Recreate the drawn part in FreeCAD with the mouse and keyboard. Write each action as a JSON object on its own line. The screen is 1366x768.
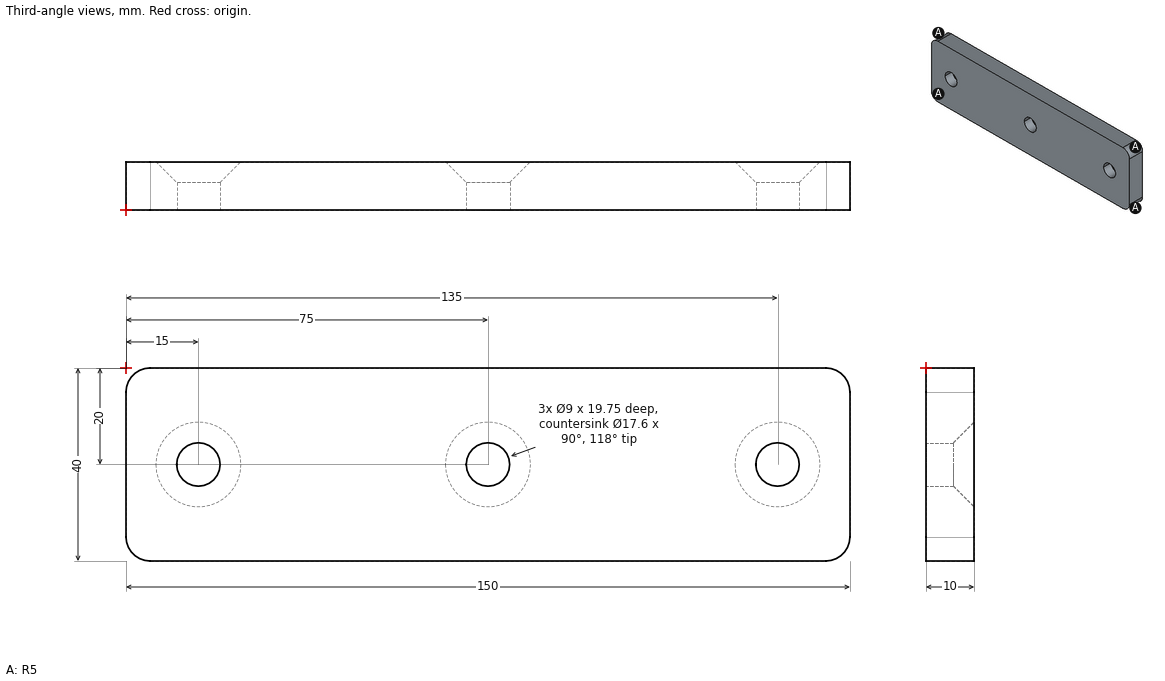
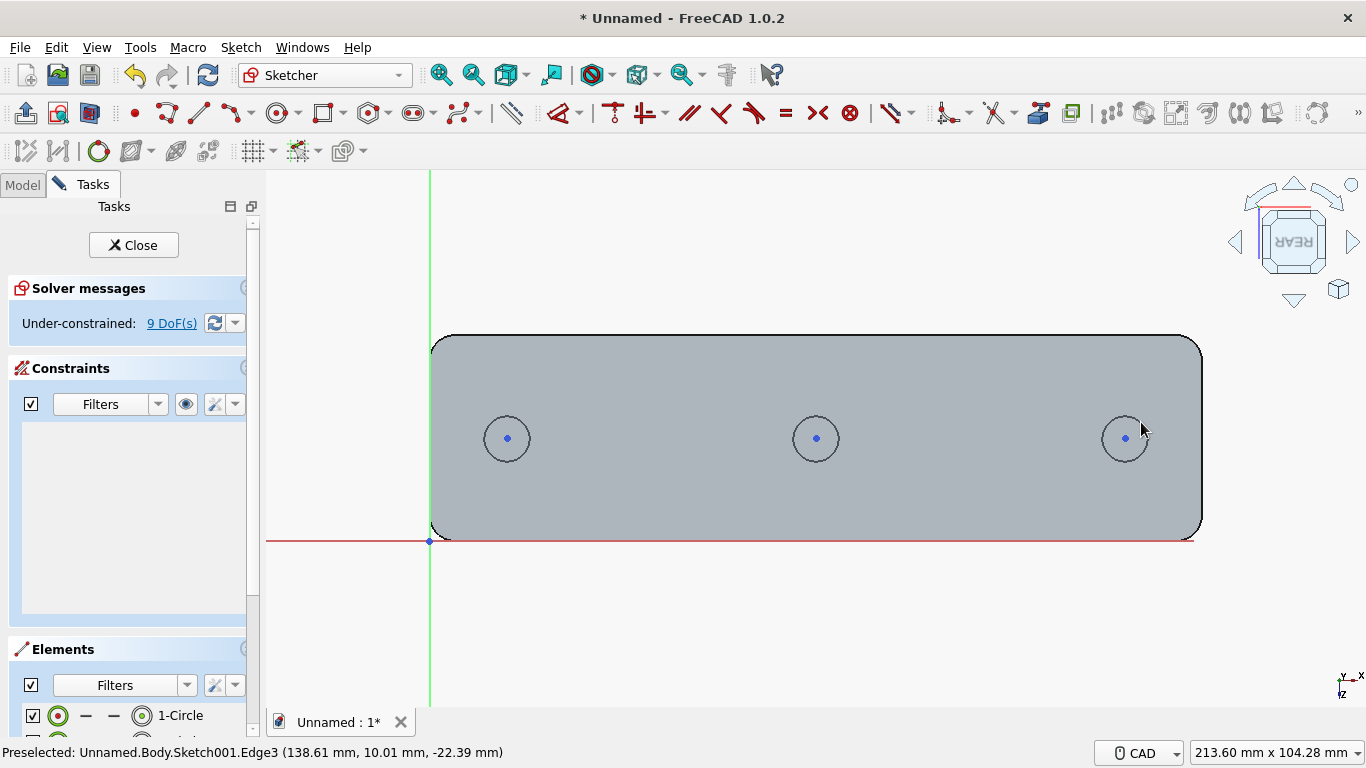
{"action": "left_click", "coordinate": [832, 423]}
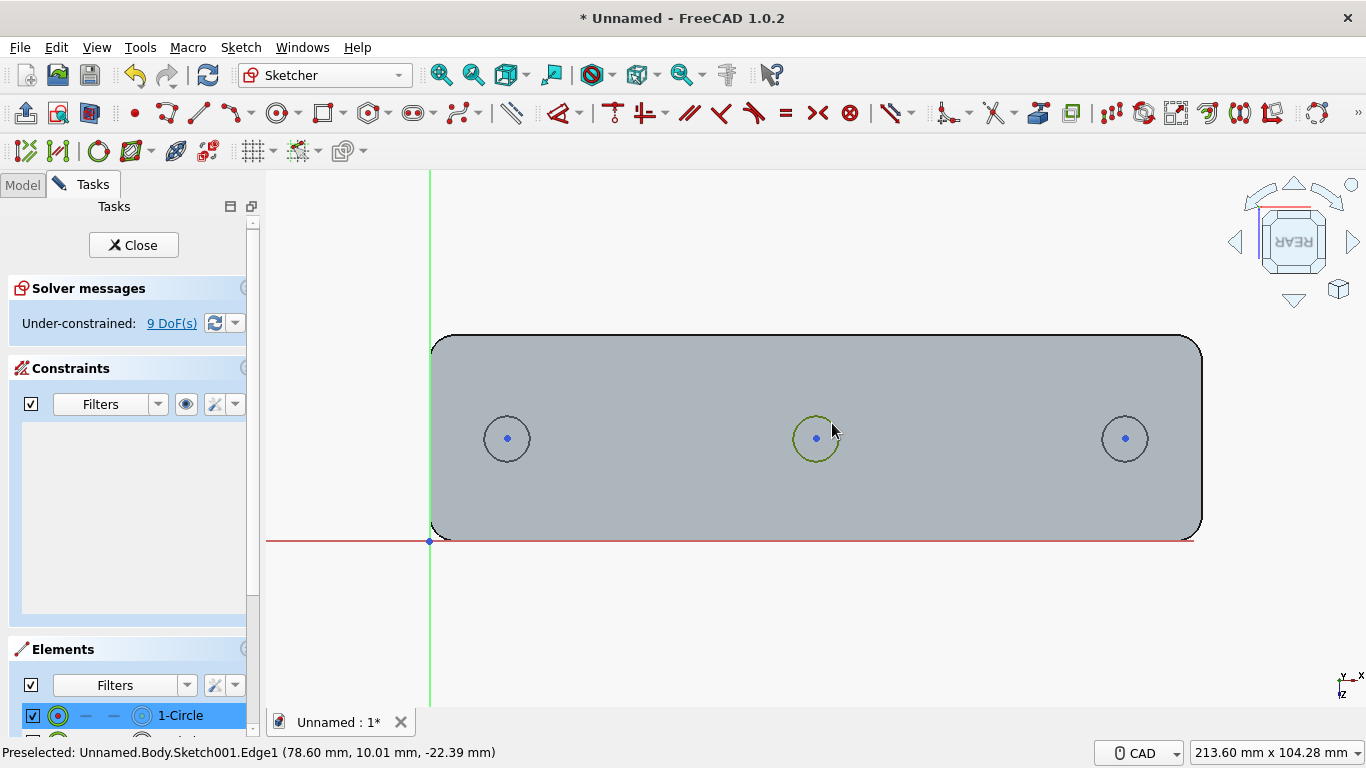
{"action": "left_click", "coordinate": [523, 423]}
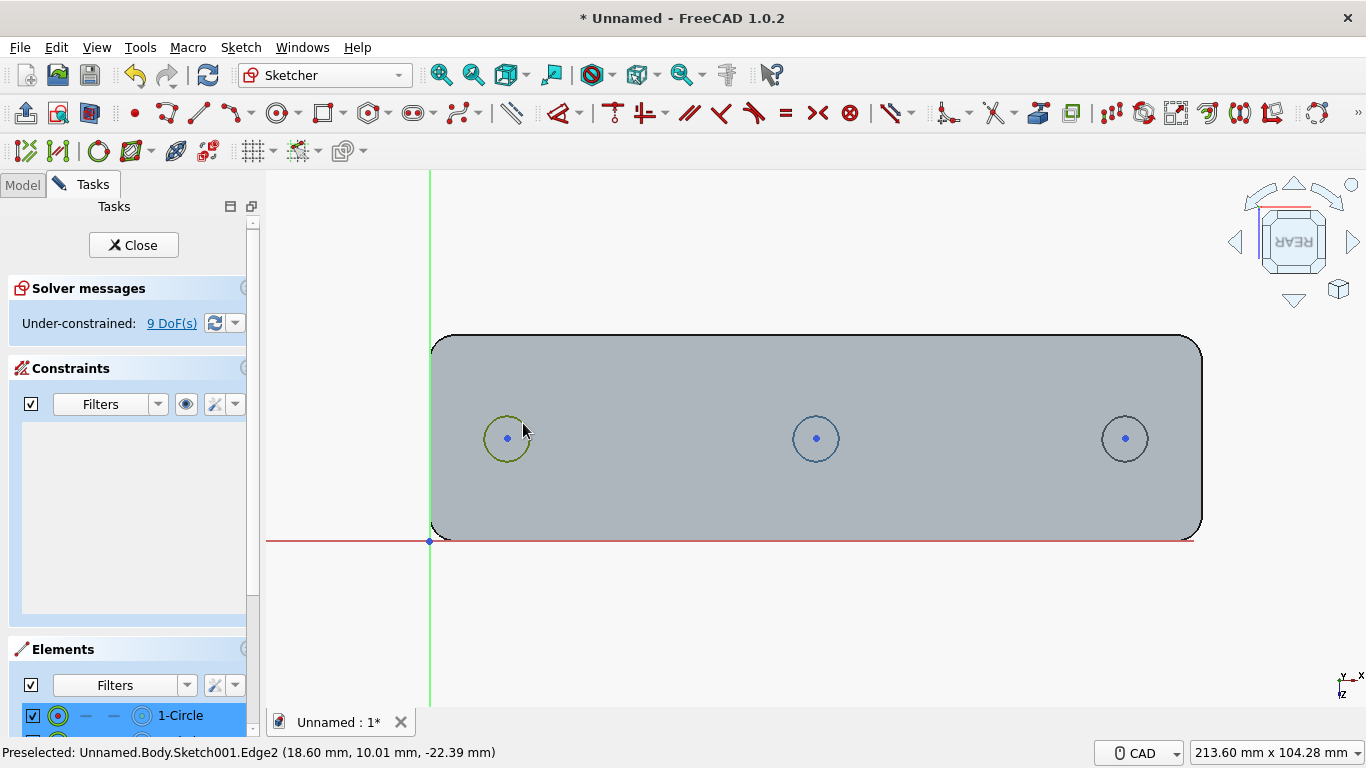
{"action": "left_click", "coordinate": [1141, 423]}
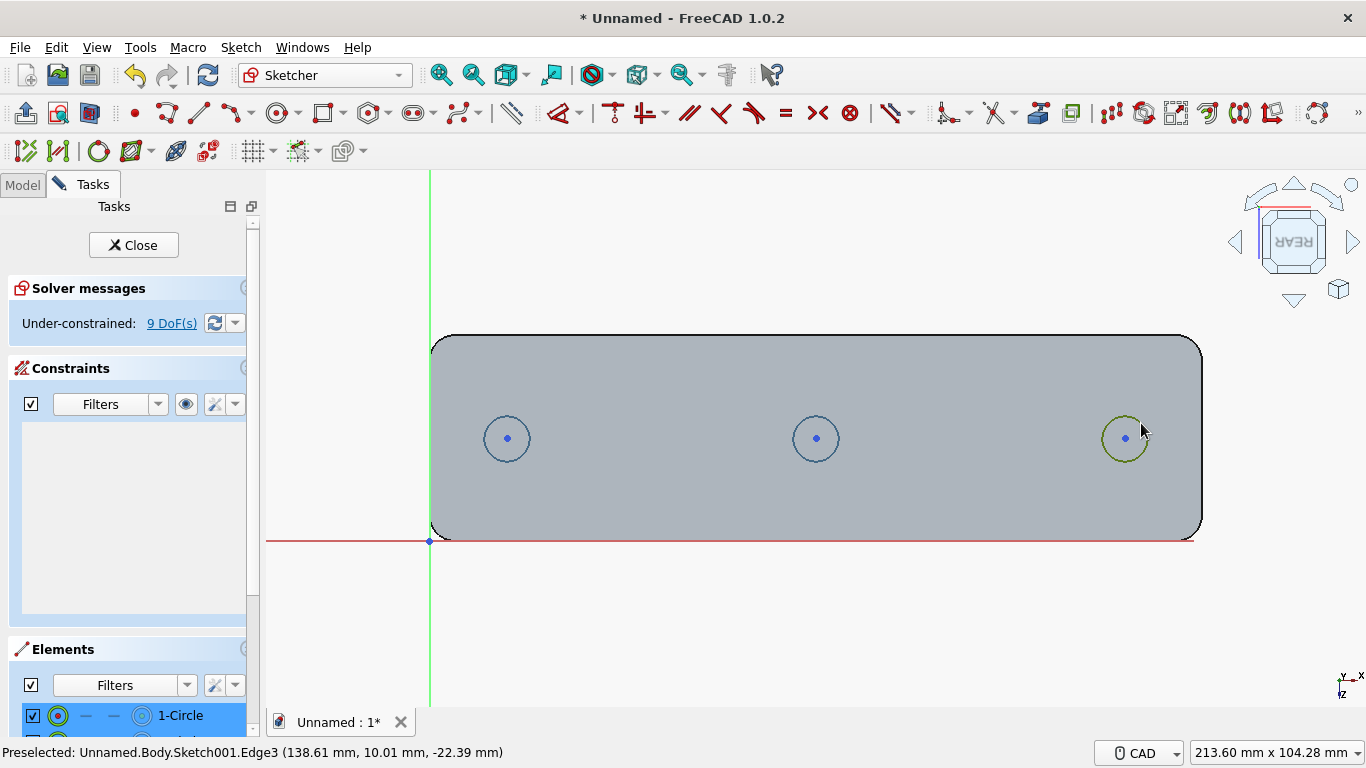
{"action": "left_click", "coordinate": [786, 114]}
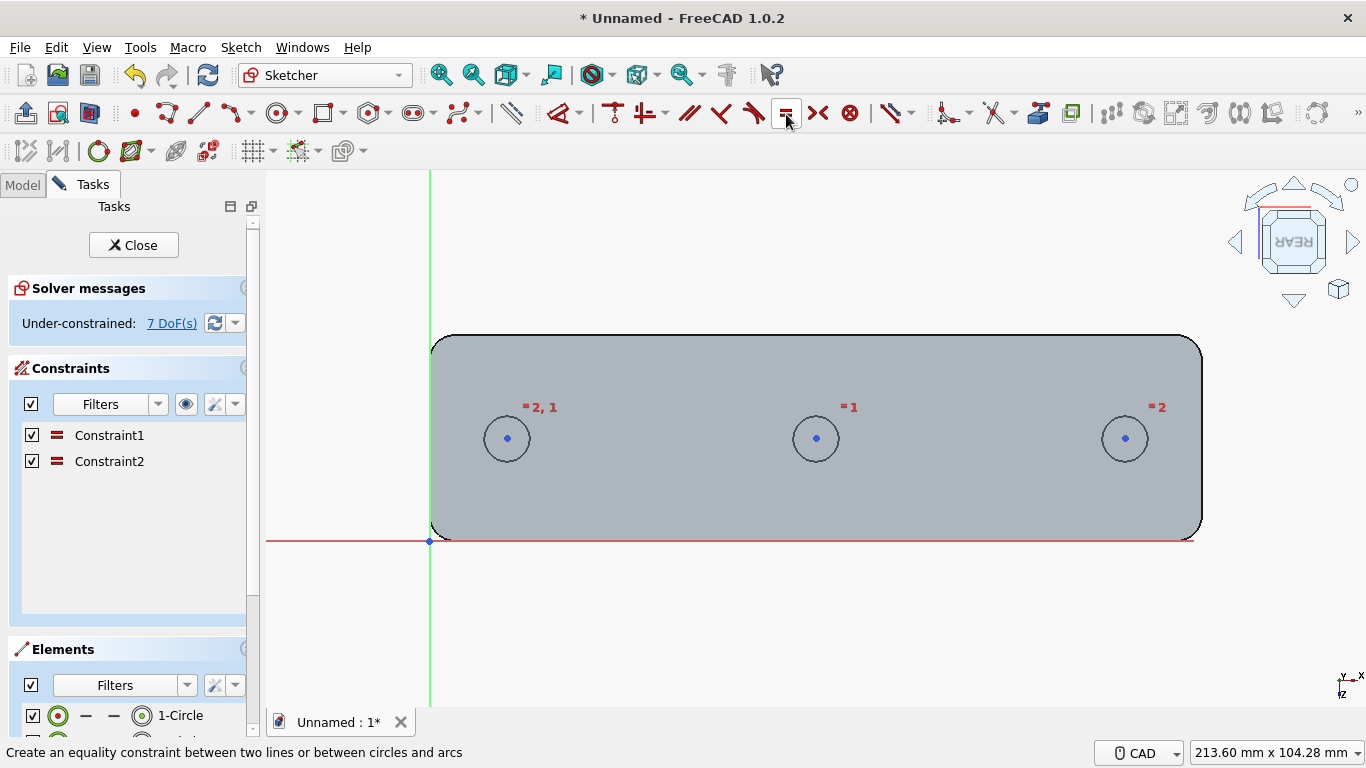
{"action": "left_click", "coordinate": [816, 439]}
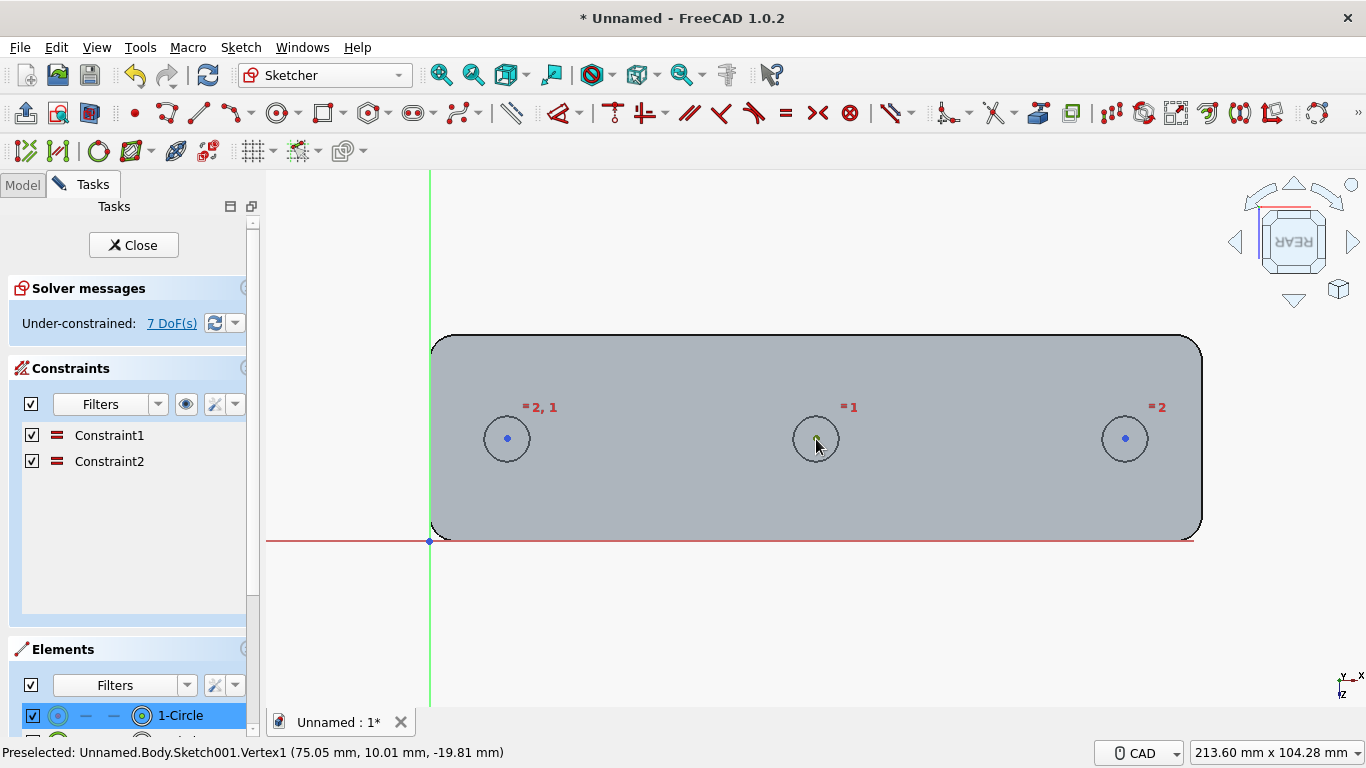
{"action": "left_click", "coordinate": [507, 439]}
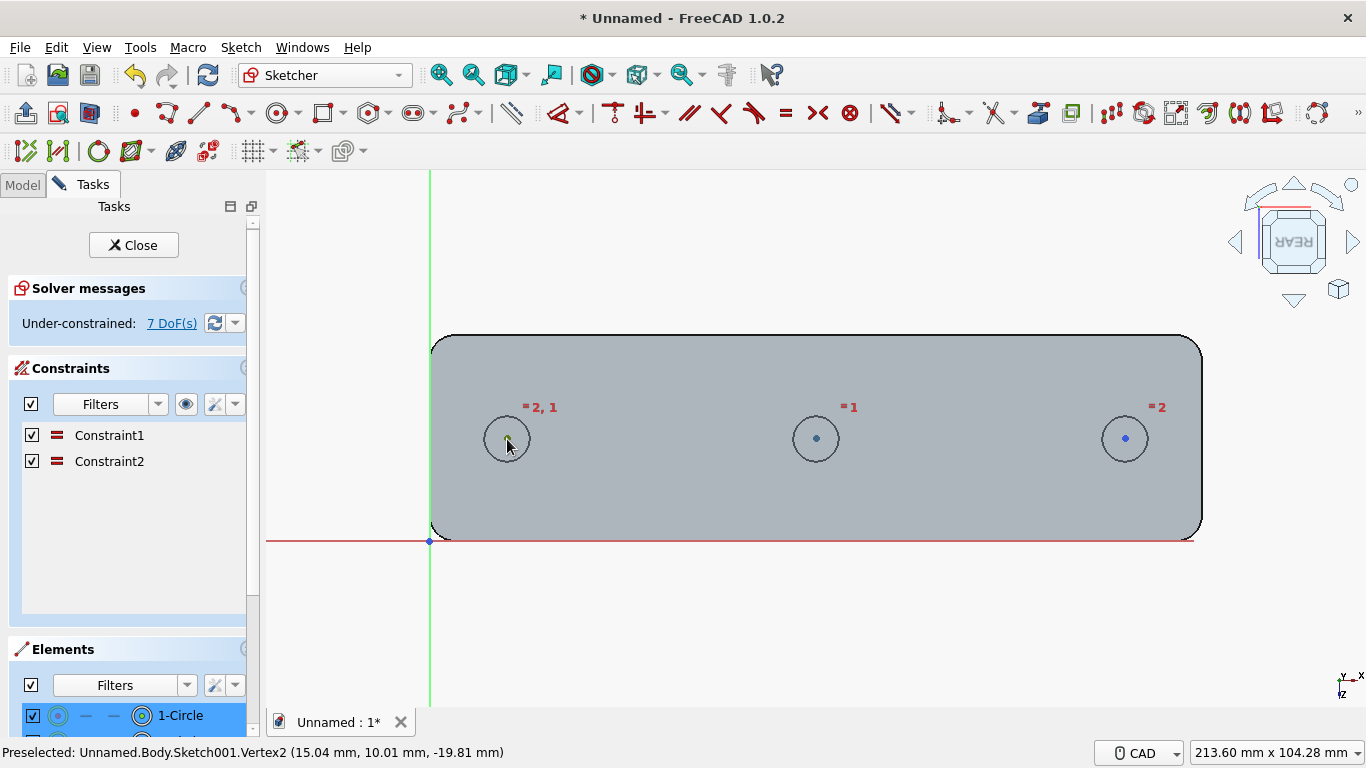
{"action": "left_click", "coordinate": [668, 114]}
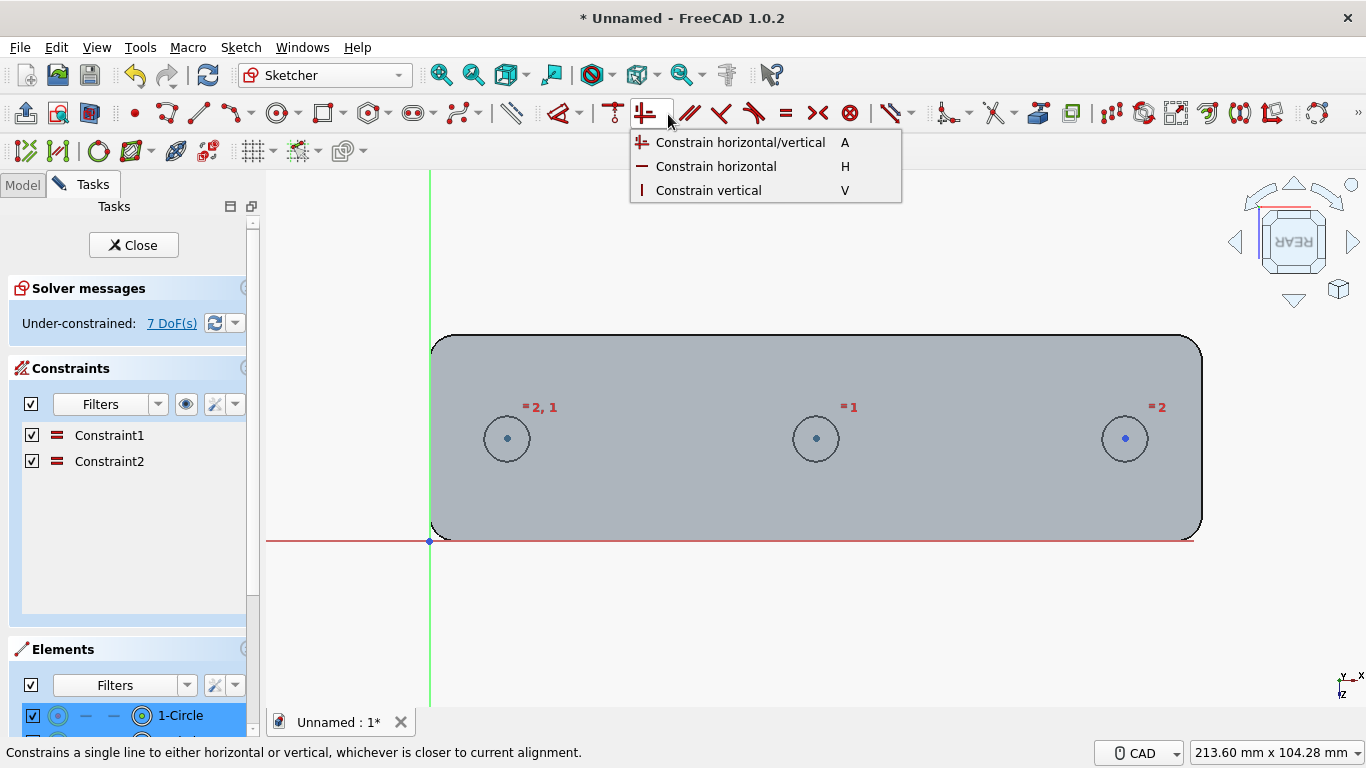
{"action": "left_click", "coordinate": [766, 166]}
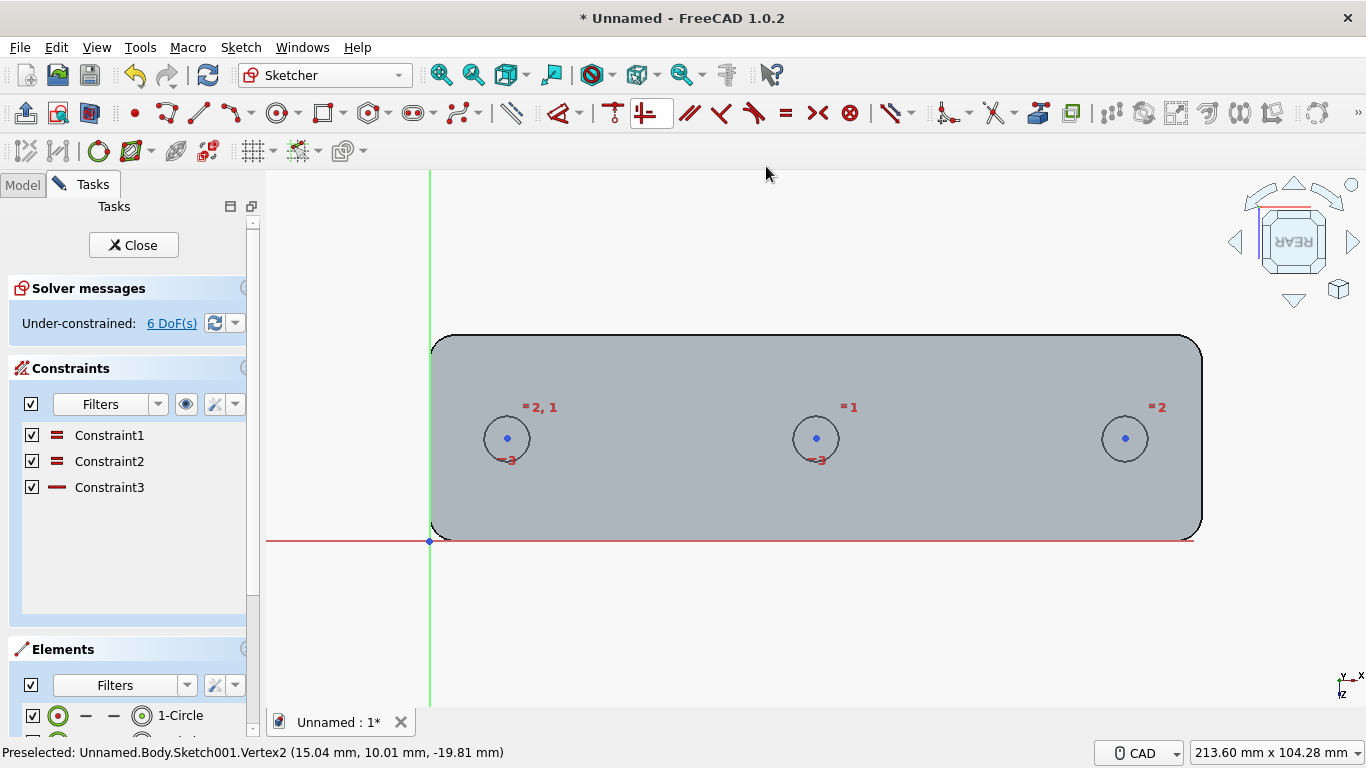
{"action": "left_click", "coordinate": [816, 439]}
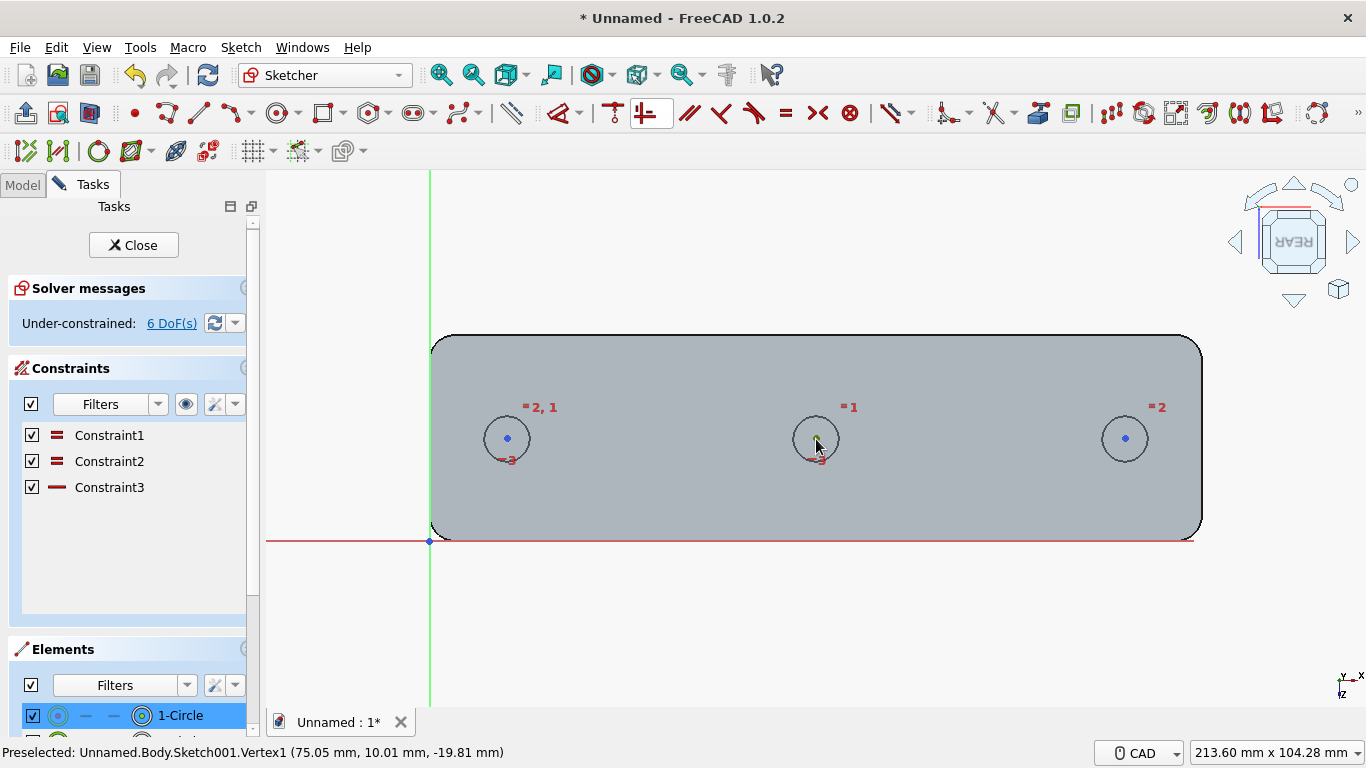
{"action": "left_click", "coordinate": [1125, 439]}